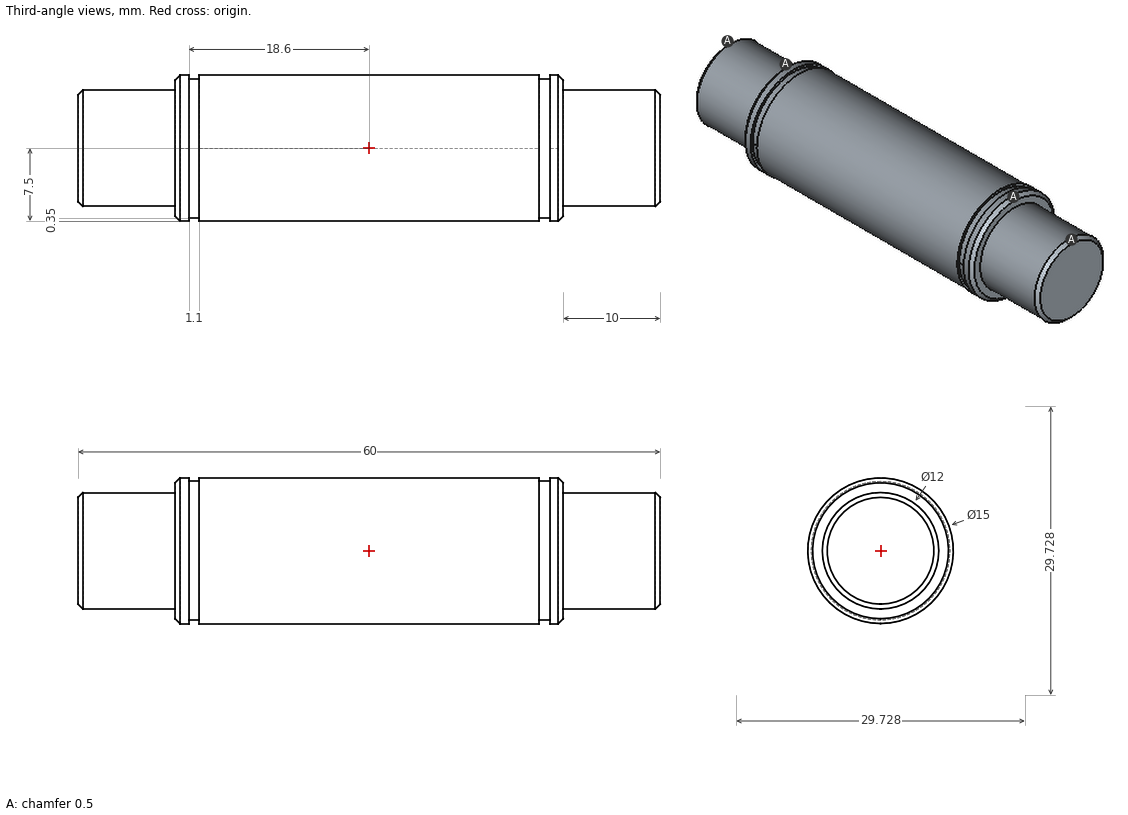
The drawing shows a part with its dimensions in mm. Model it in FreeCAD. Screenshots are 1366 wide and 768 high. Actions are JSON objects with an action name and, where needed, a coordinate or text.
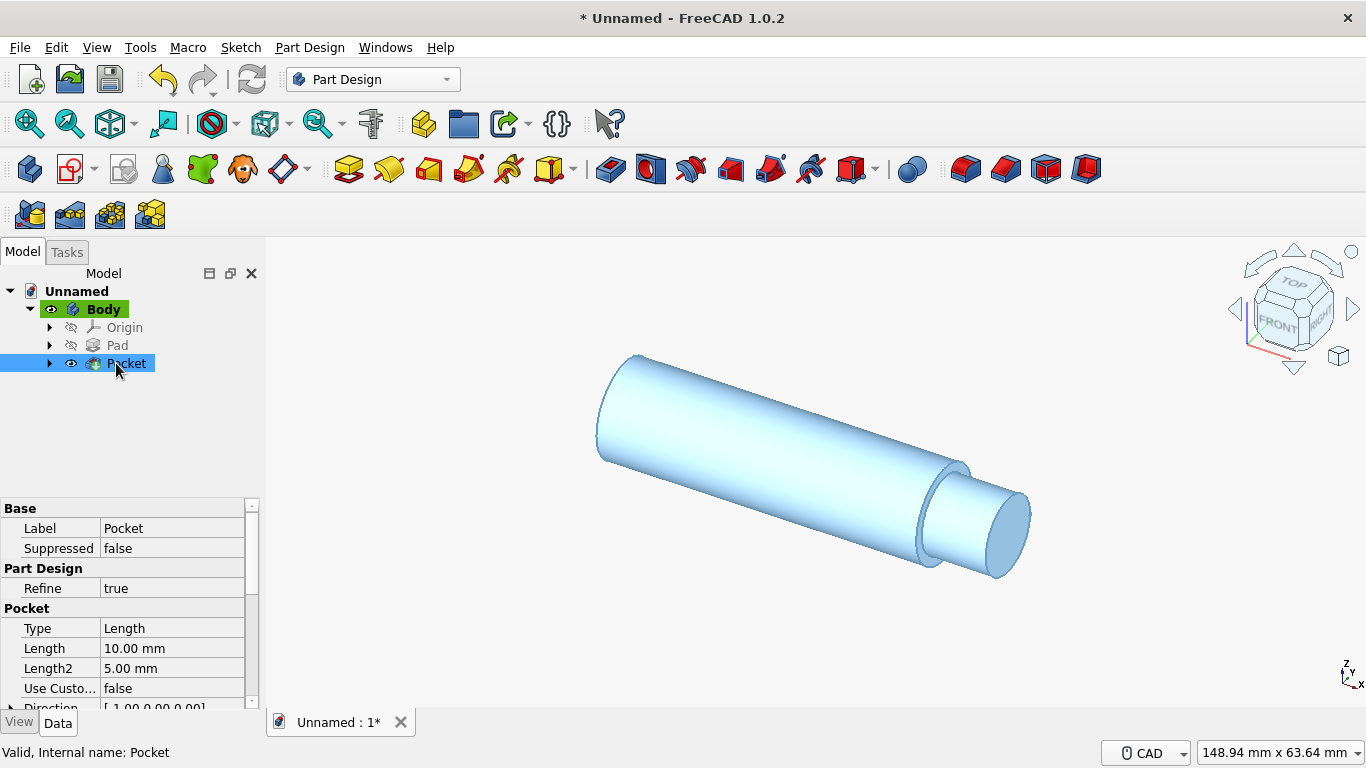
{"action": "left_click", "coordinate": [30, 214]}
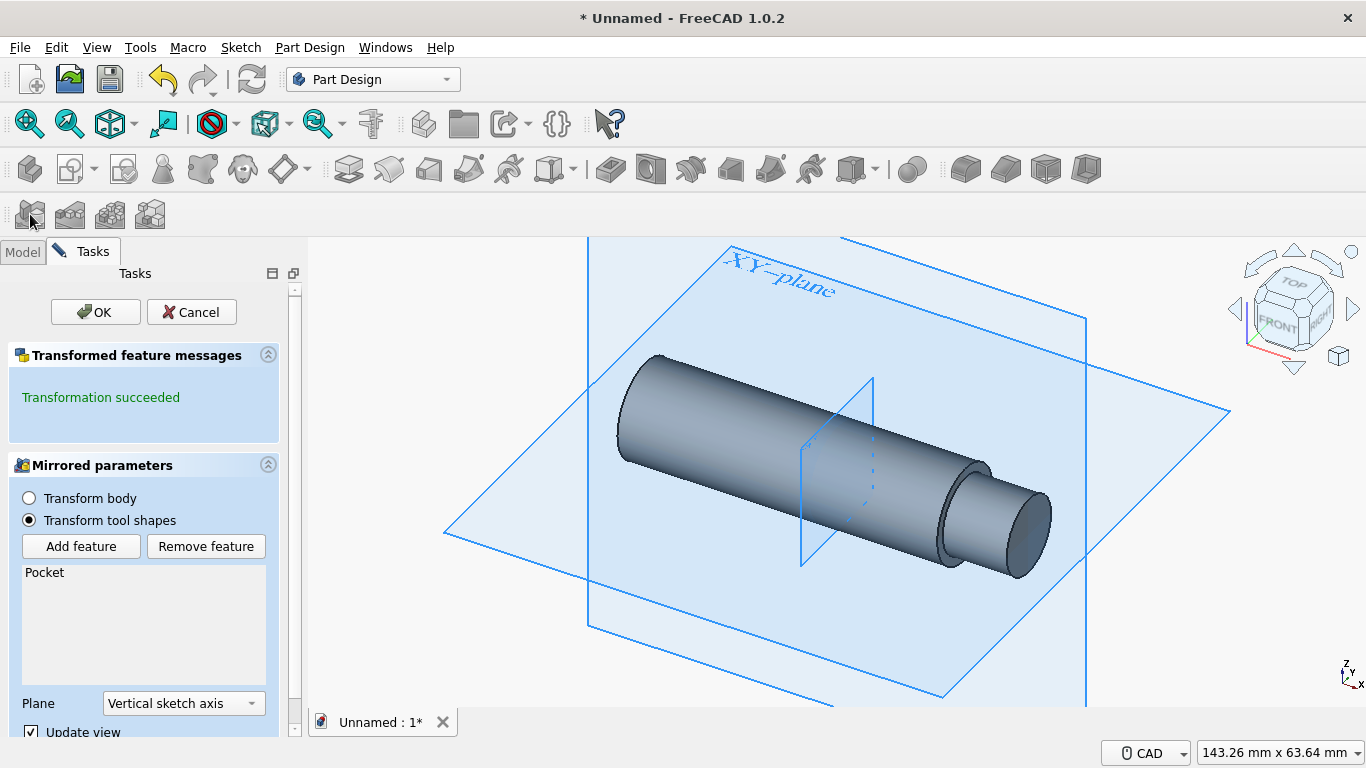
{"action": "left_click", "coordinate": [184, 704]}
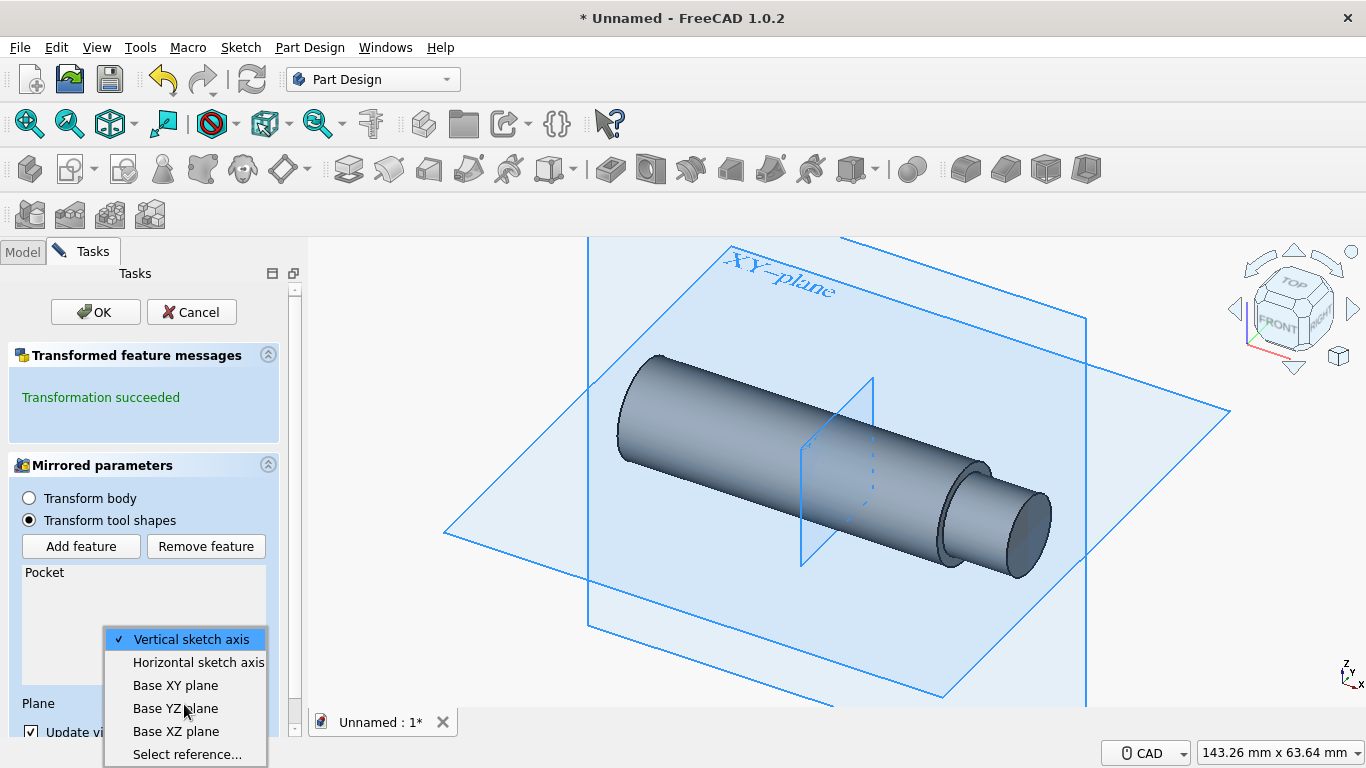
{"action": "left_click", "coordinate": [184, 708]}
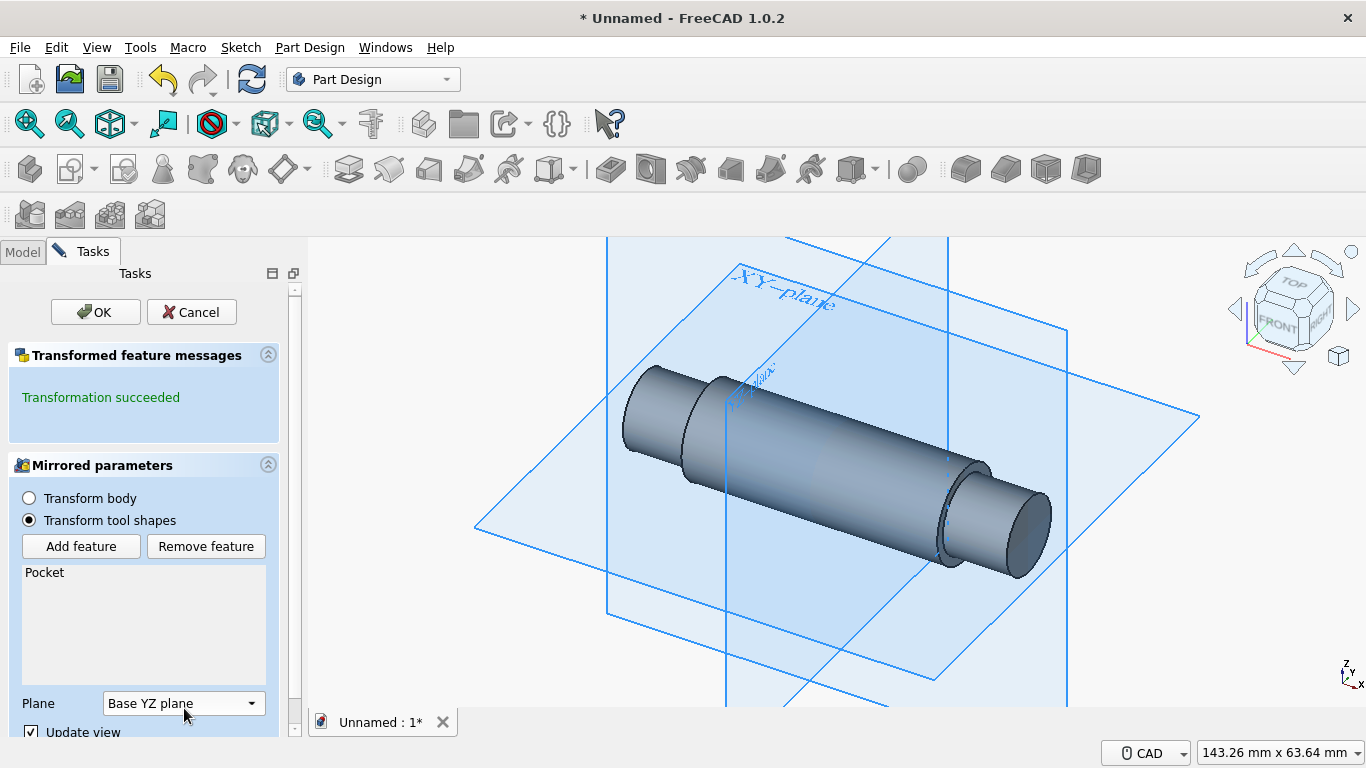
{"action": "left_click", "coordinate": [96, 312]}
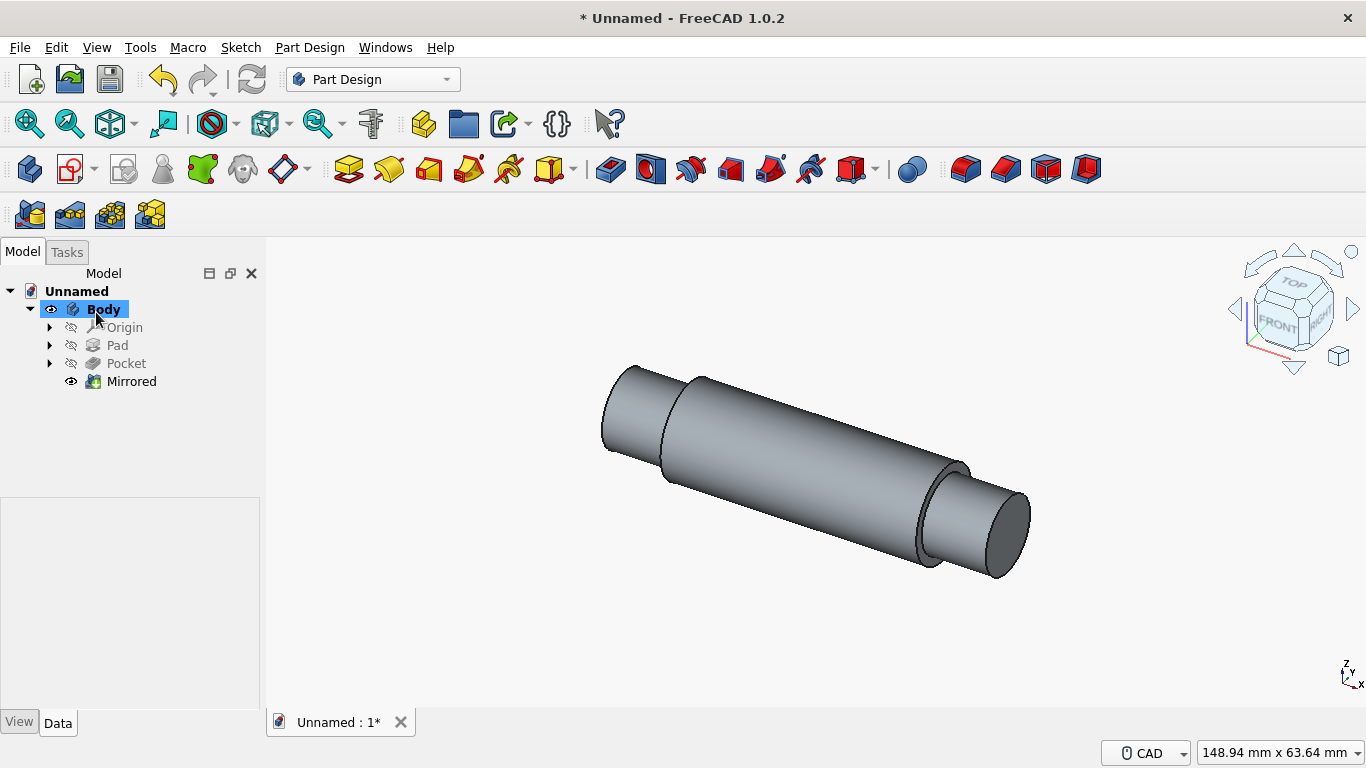
{"action": "left_click", "coordinate": [986, 557]}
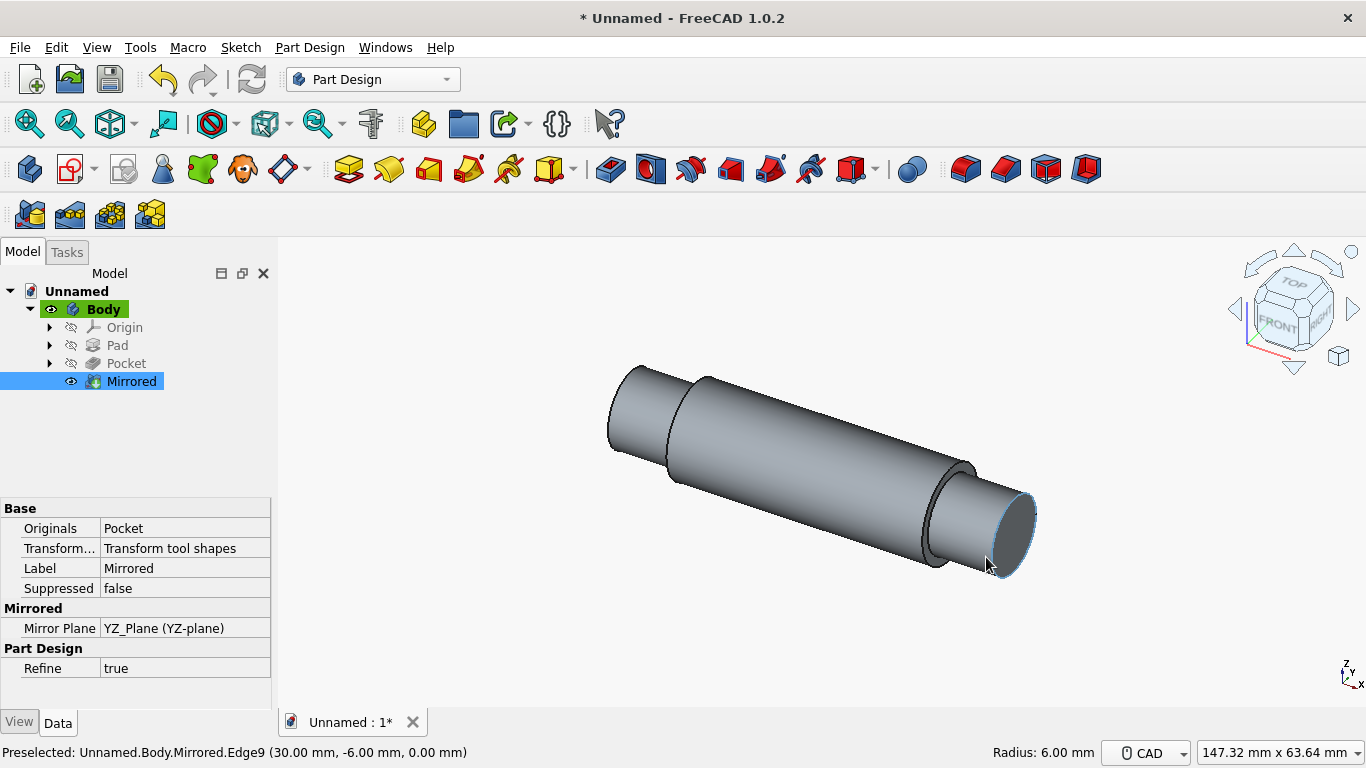
{"action": "left_click", "coordinate": [623, 380], "text": "ctrl"}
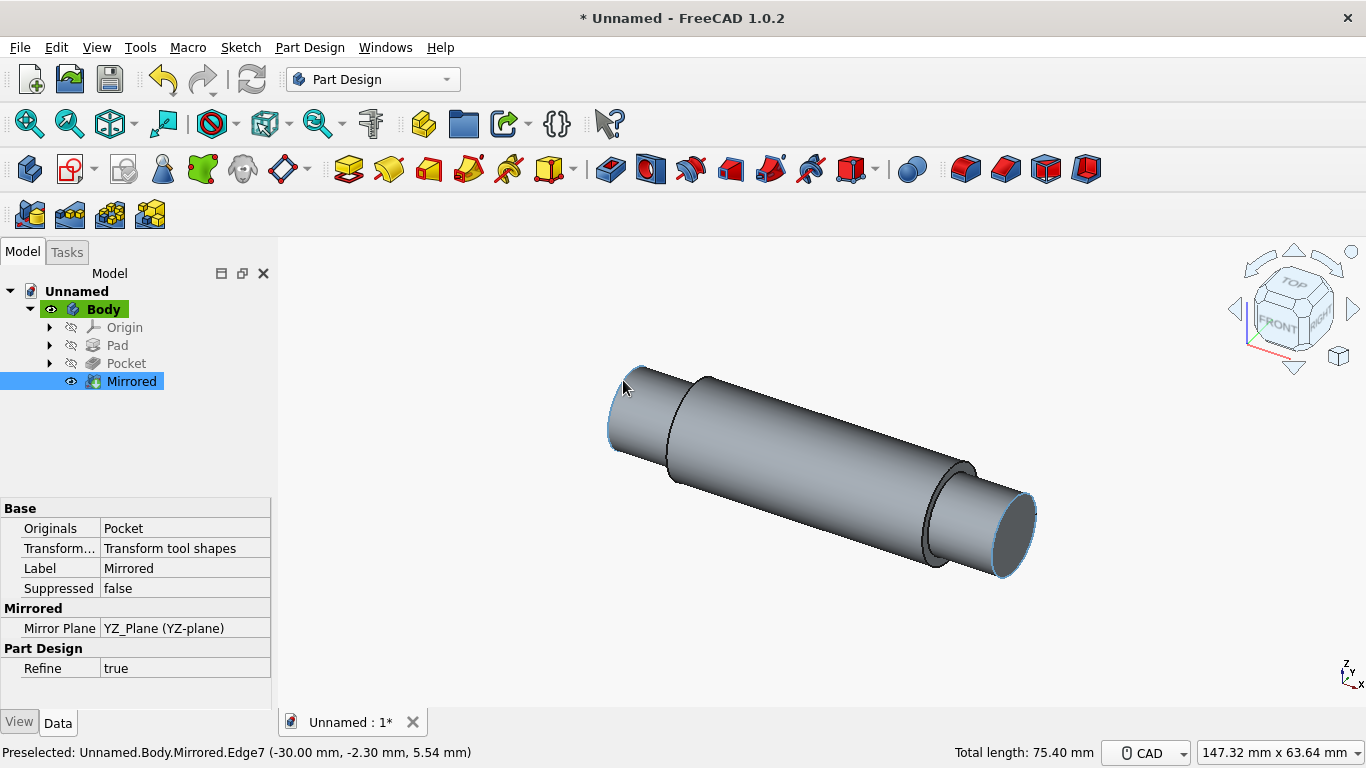
{"action": "left_click", "coordinate": [922, 541], "text": "ctrl"}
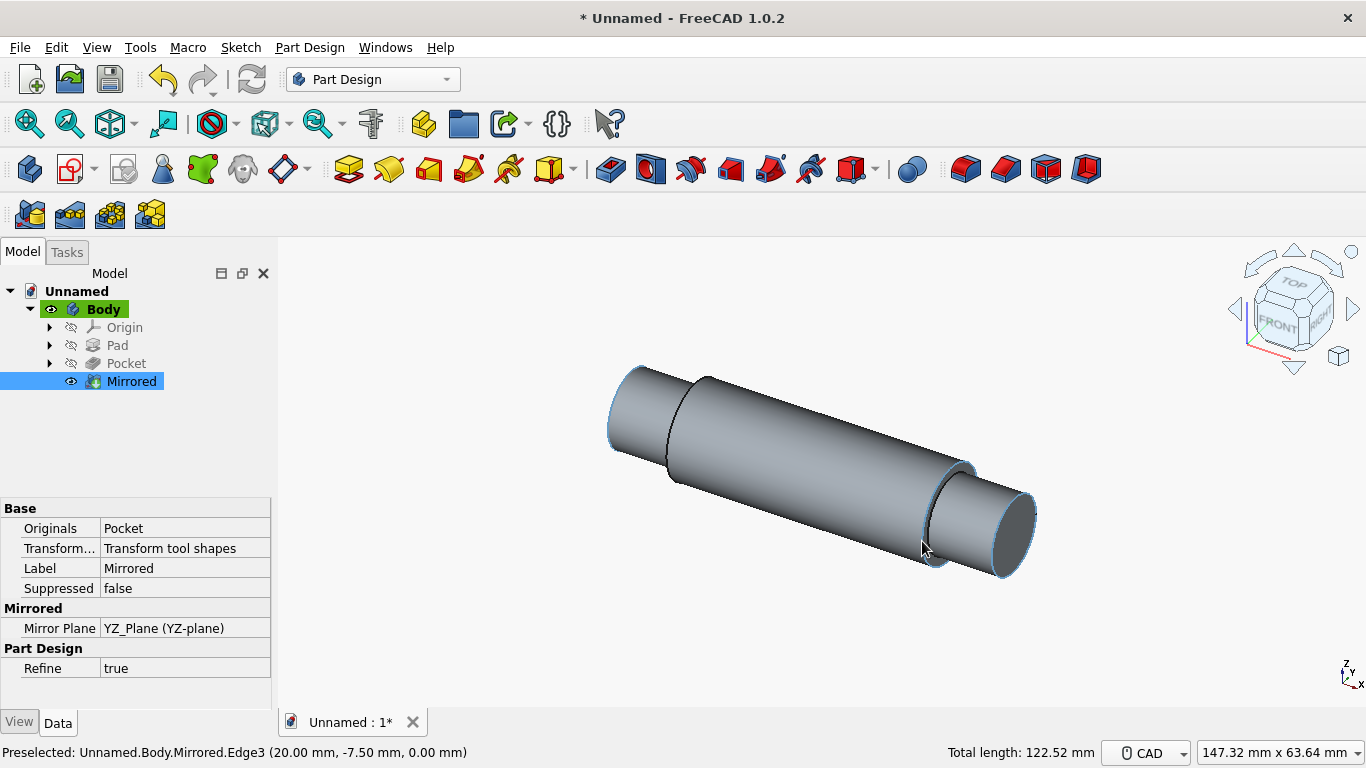
{"action": "key", "text": "0"}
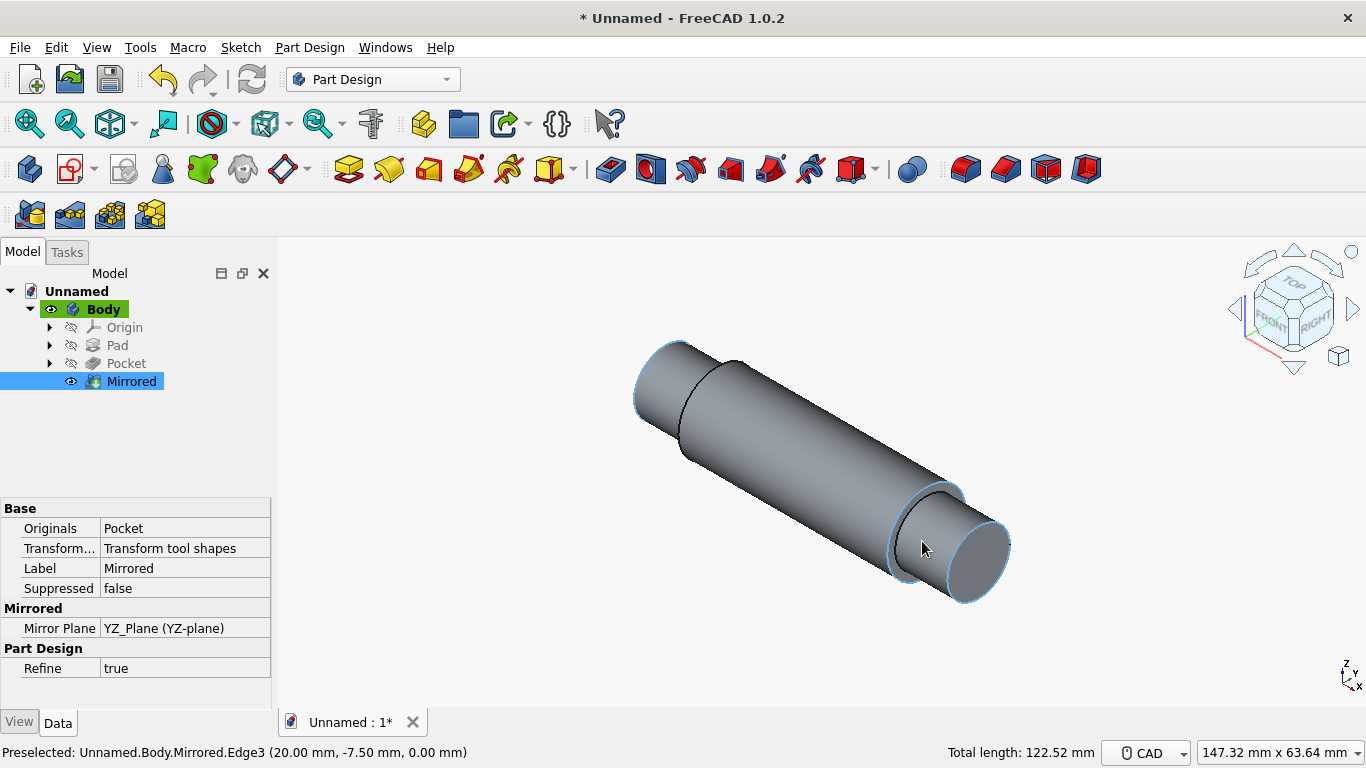
{"action": "key", "text": "2"}